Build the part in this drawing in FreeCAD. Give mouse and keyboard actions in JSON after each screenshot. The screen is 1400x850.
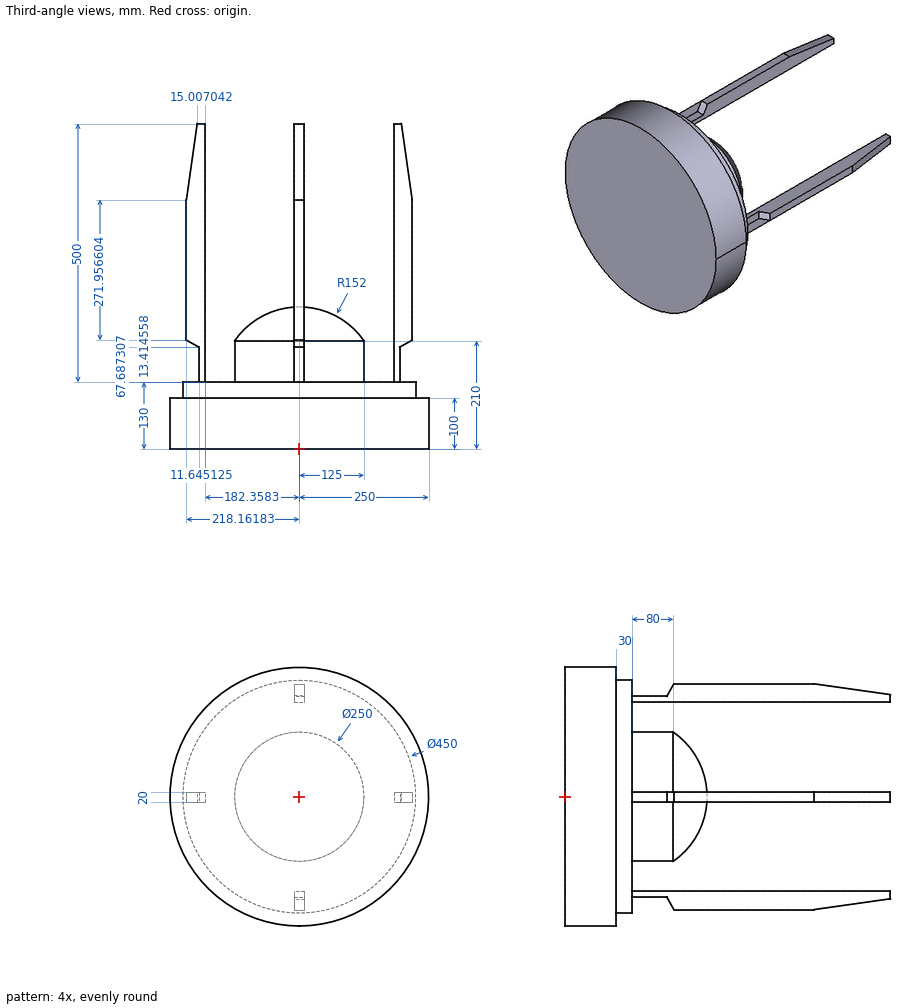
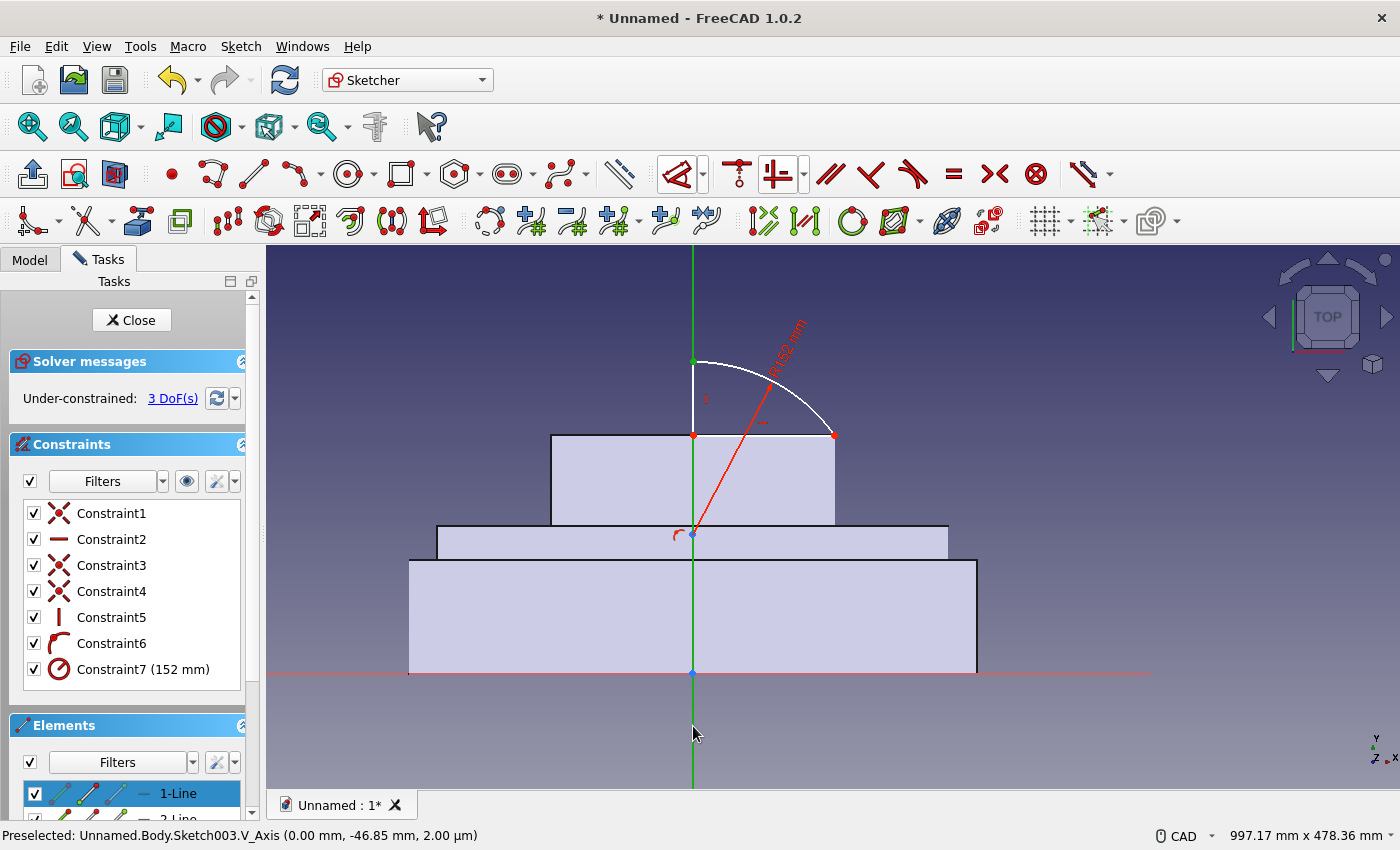
{"action": "left_click", "coordinate": [737, 174]}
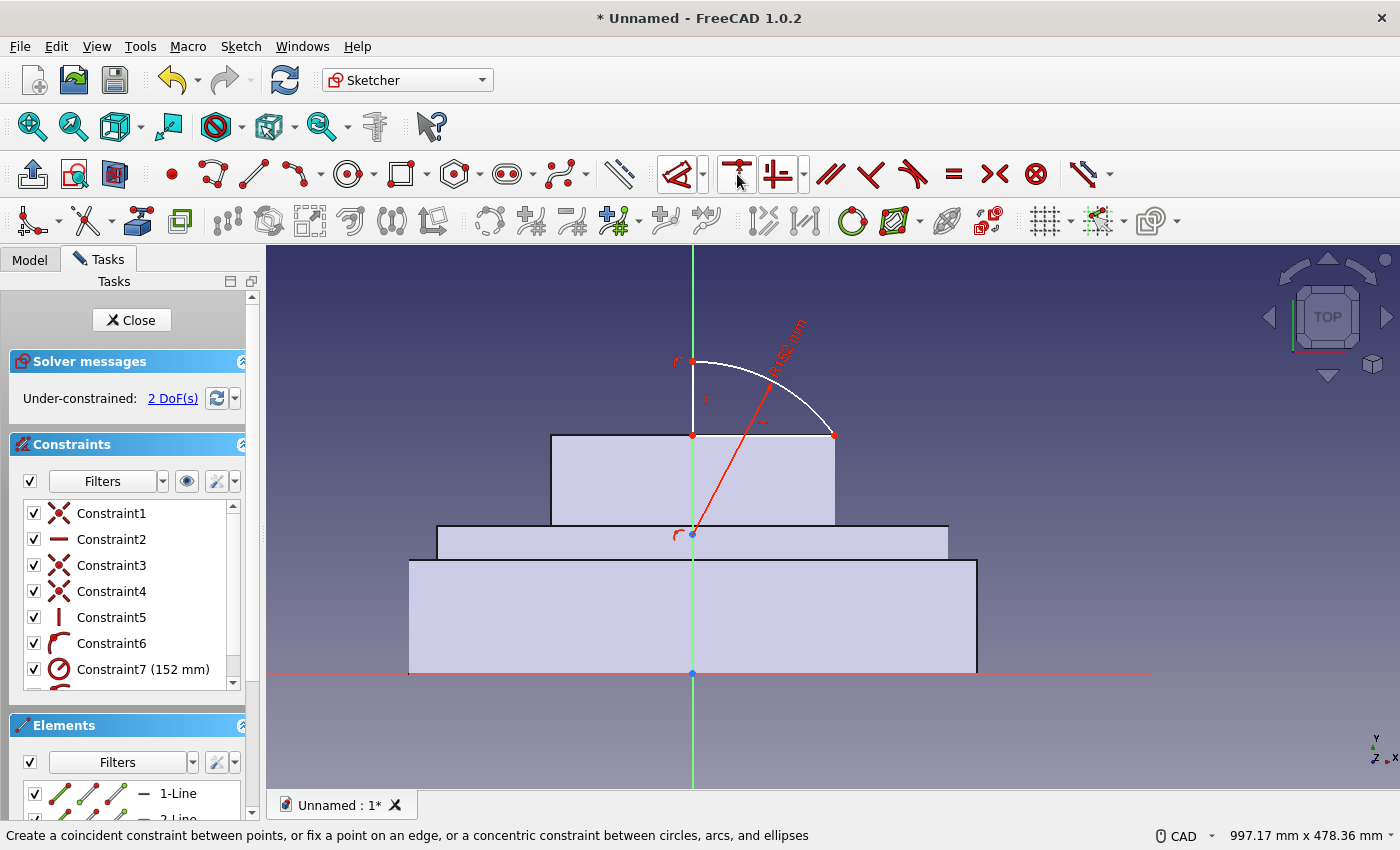
{"action": "left_click", "coordinate": [736, 436]}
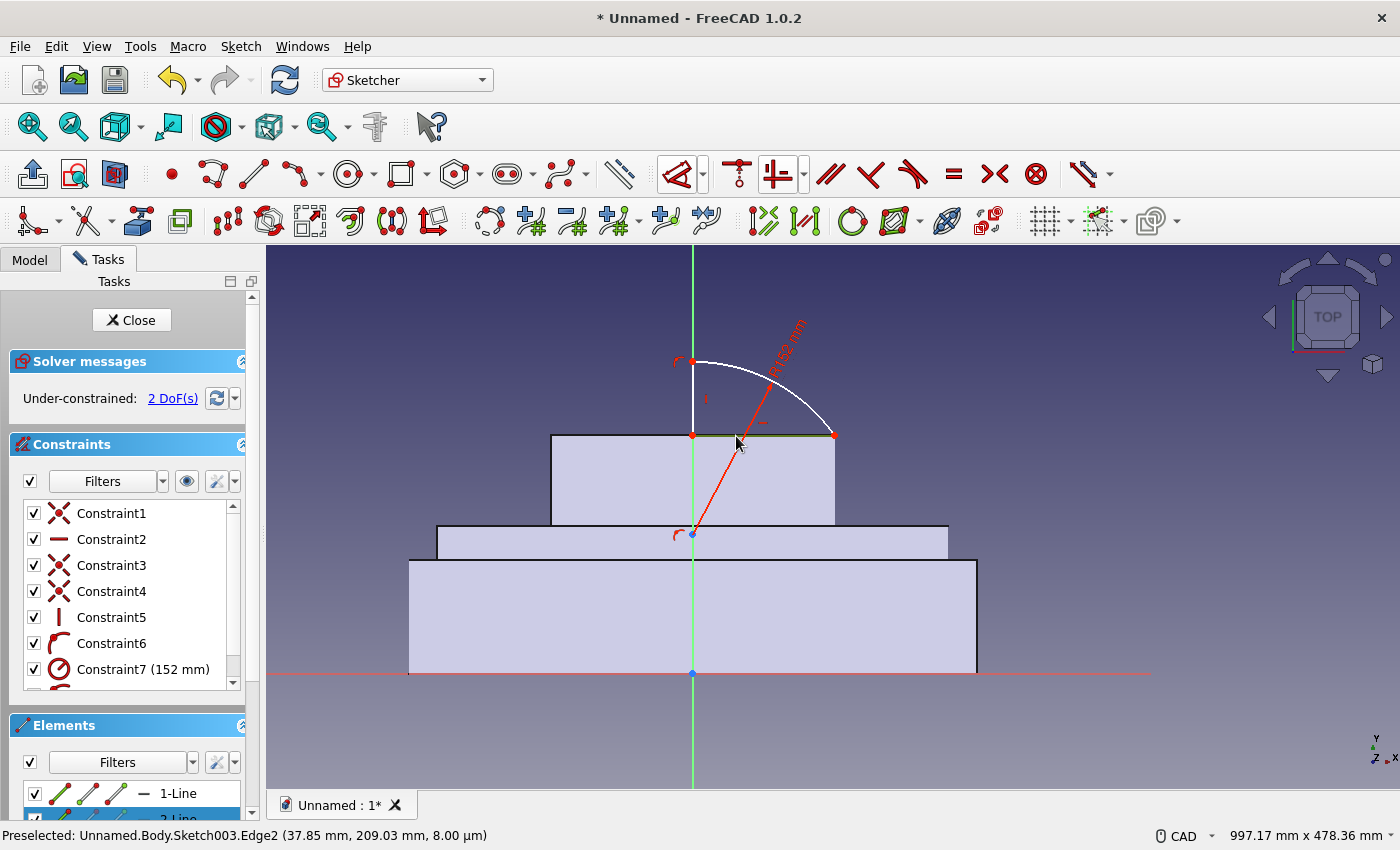
{"action": "key", "text": "l"}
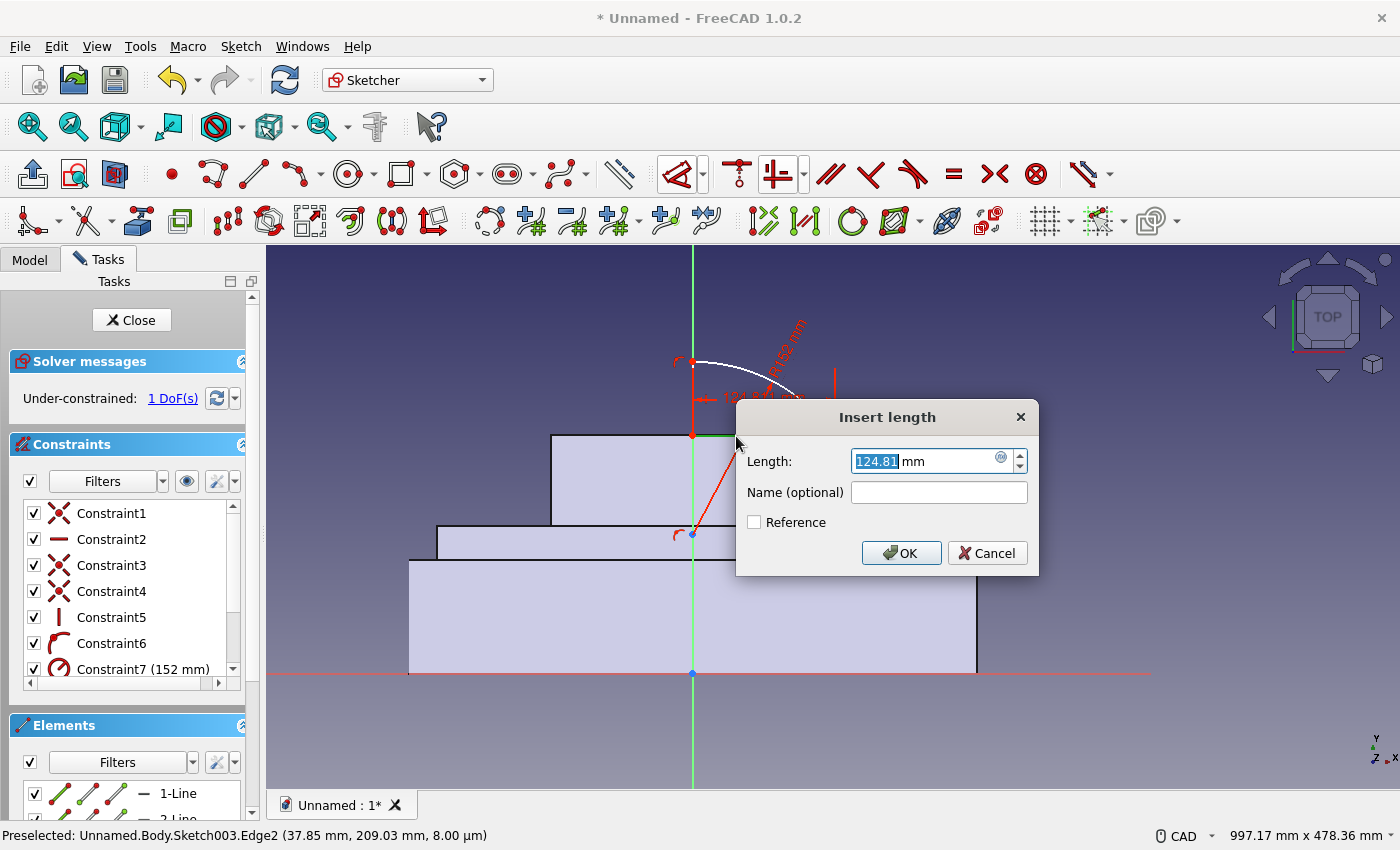
{"action": "type", "text": "125"}
{"action": "key", "text": "Return"}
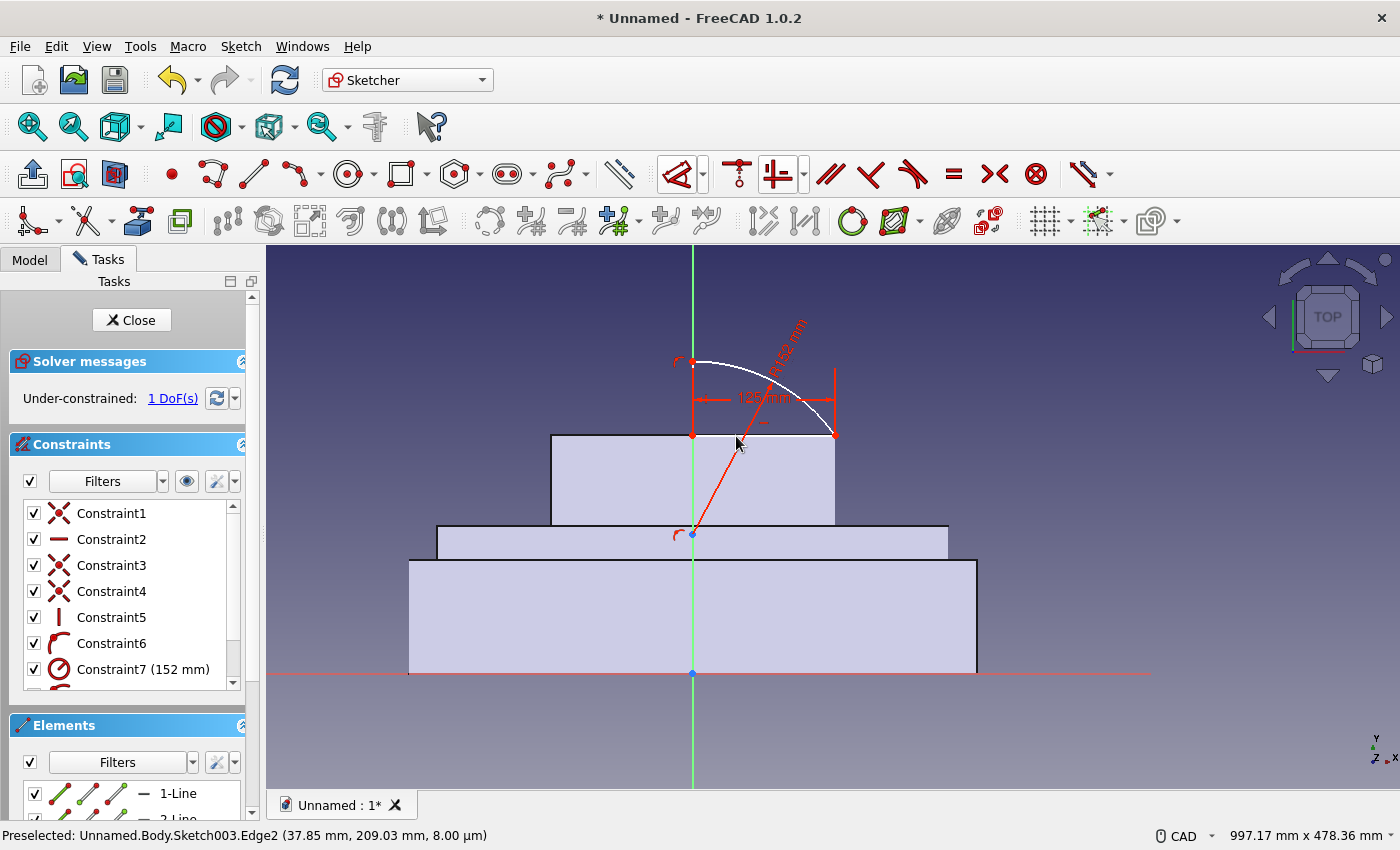
{"action": "left_click", "coordinate": [693, 436]}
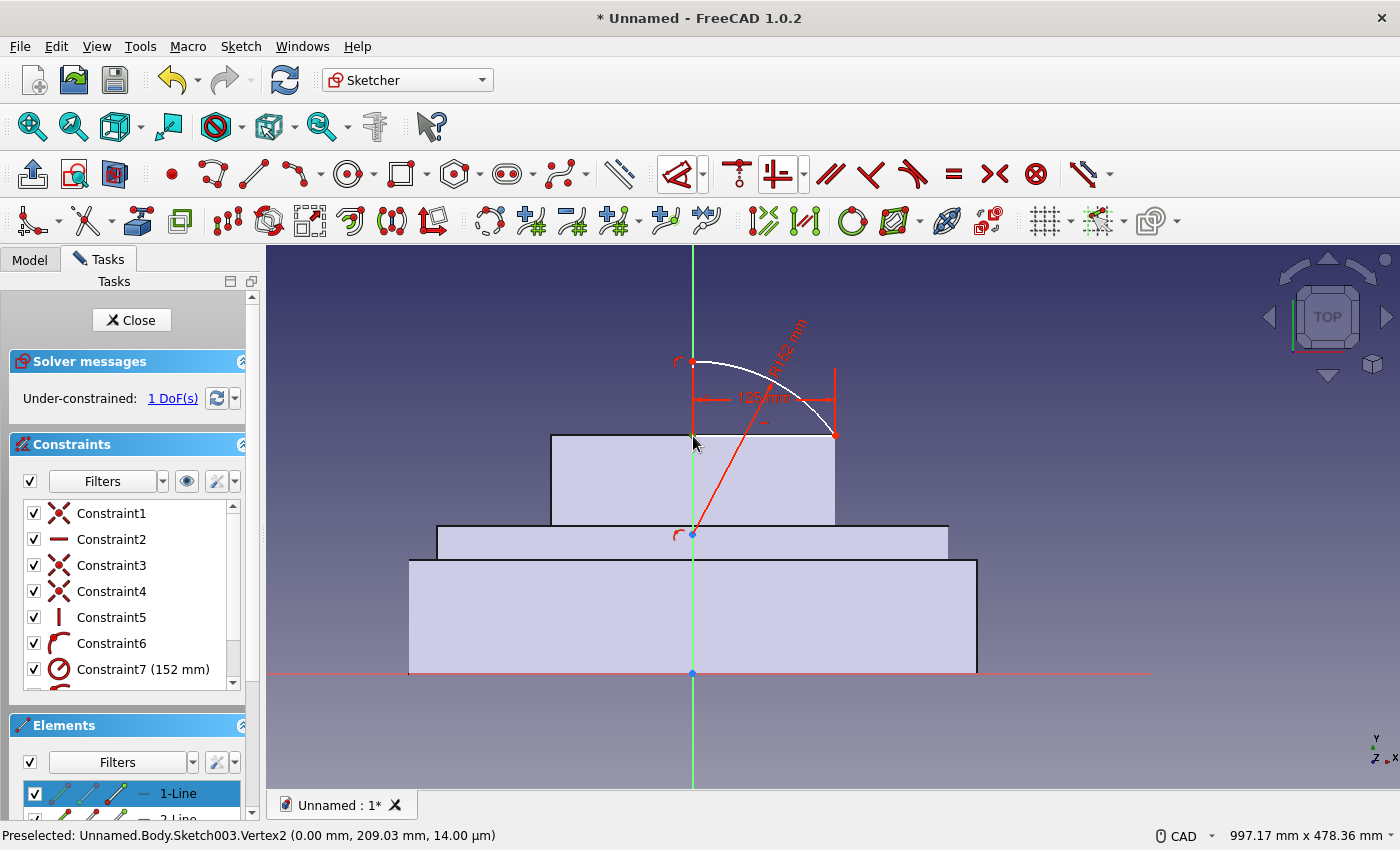
{"action": "left_click", "coordinate": [702, 174]}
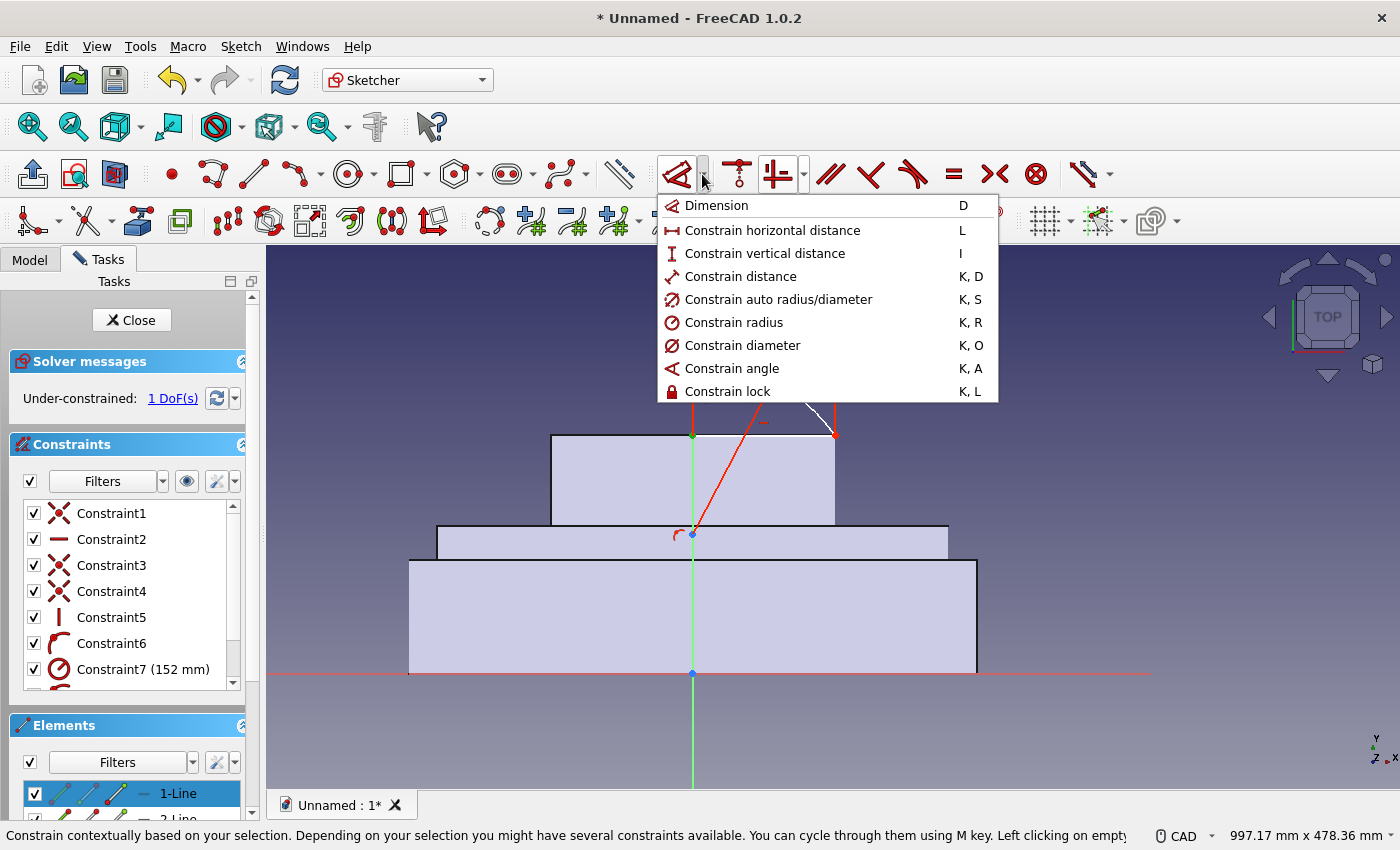
{"action": "left_click", "coordinate": [828, 254]}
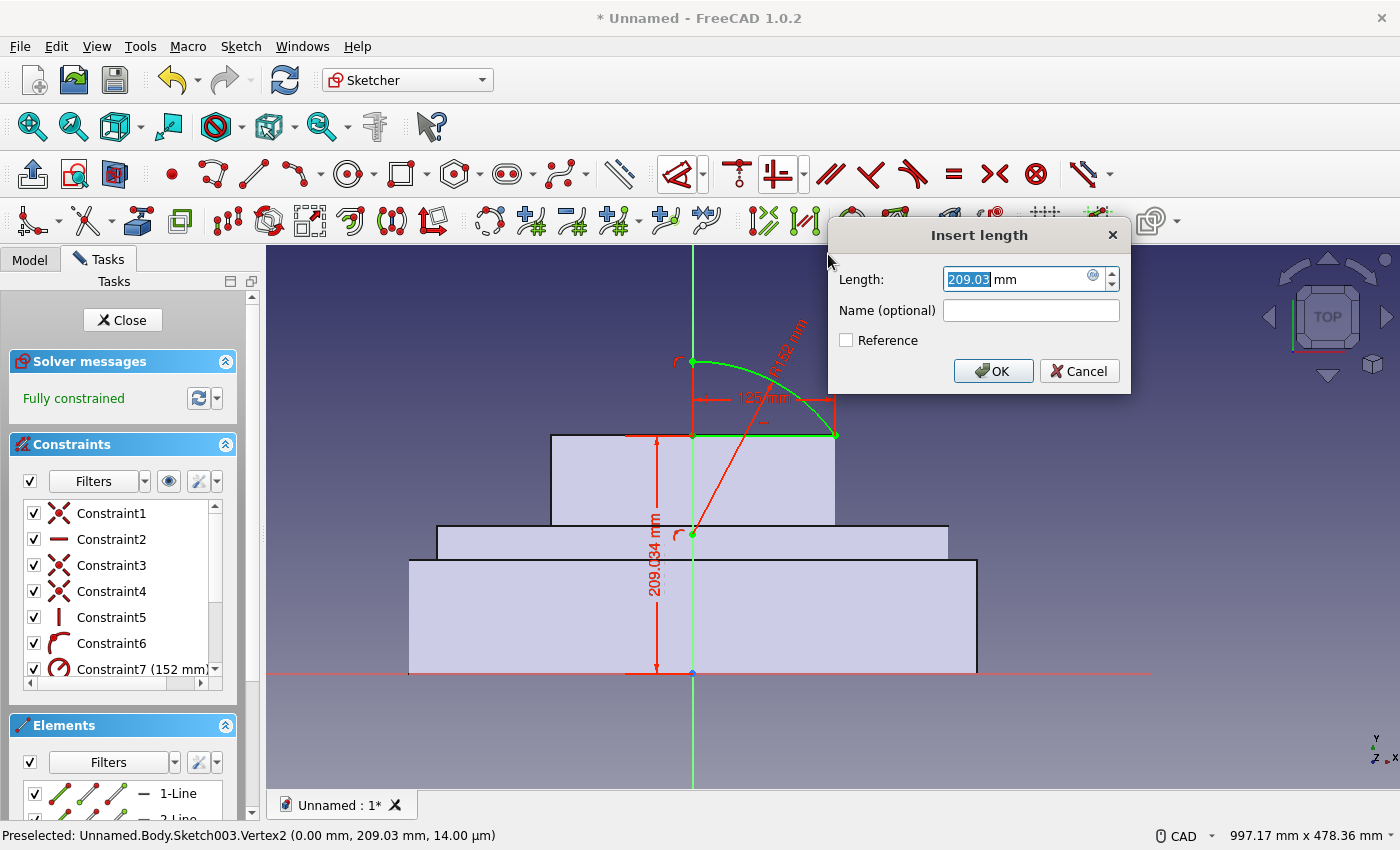
{"action": "type", "text": "210"}
{"action": "key", "text": "Return"}